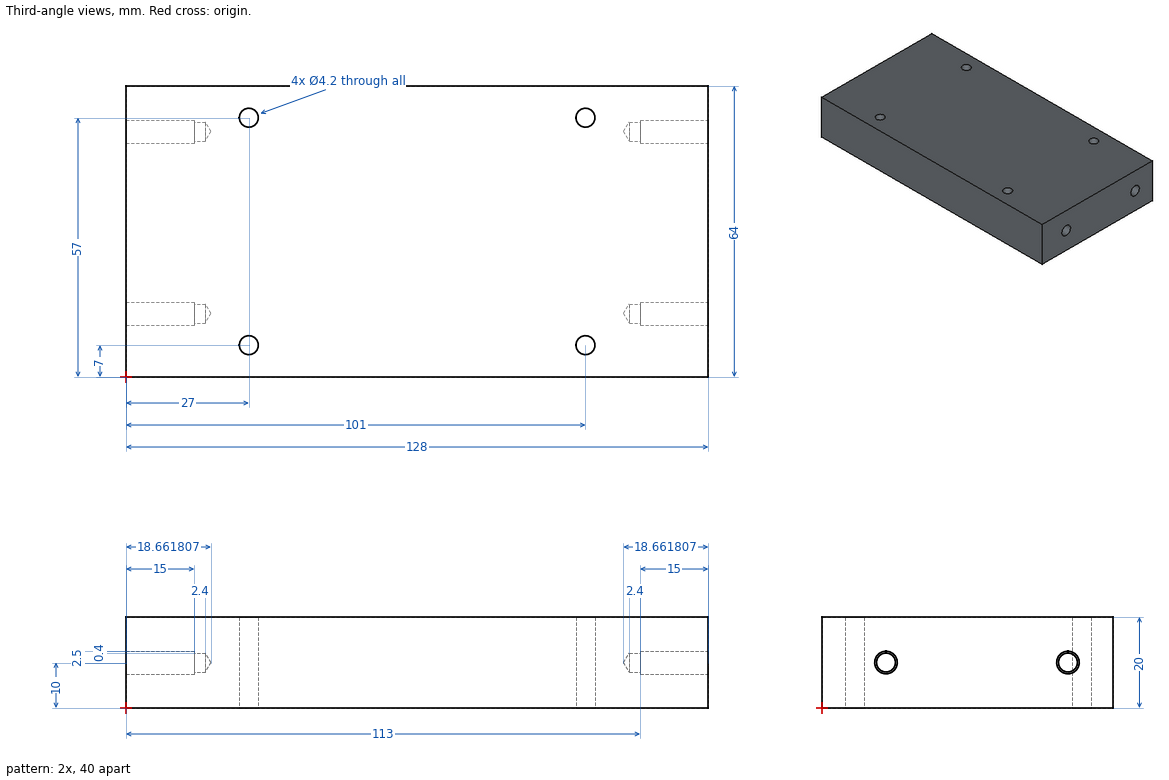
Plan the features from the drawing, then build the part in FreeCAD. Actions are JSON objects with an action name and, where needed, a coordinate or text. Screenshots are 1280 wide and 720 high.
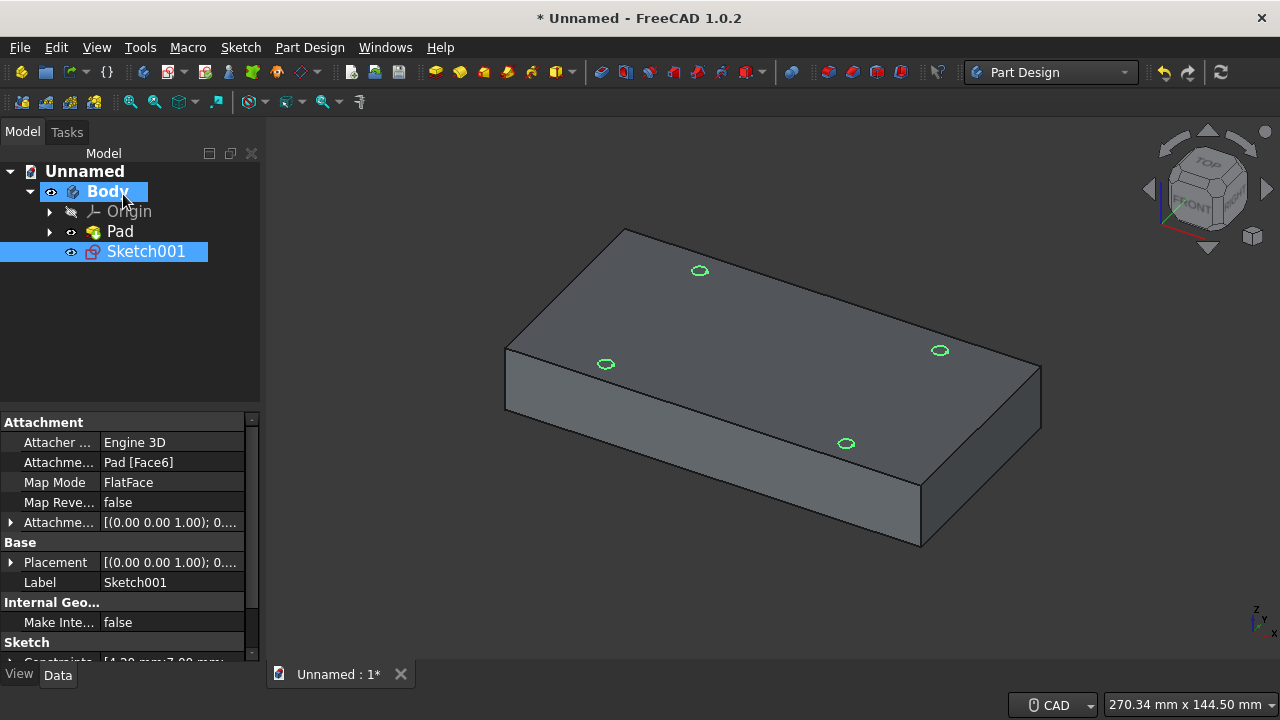
{"action": "left_click", "coordinate": [626, 72]}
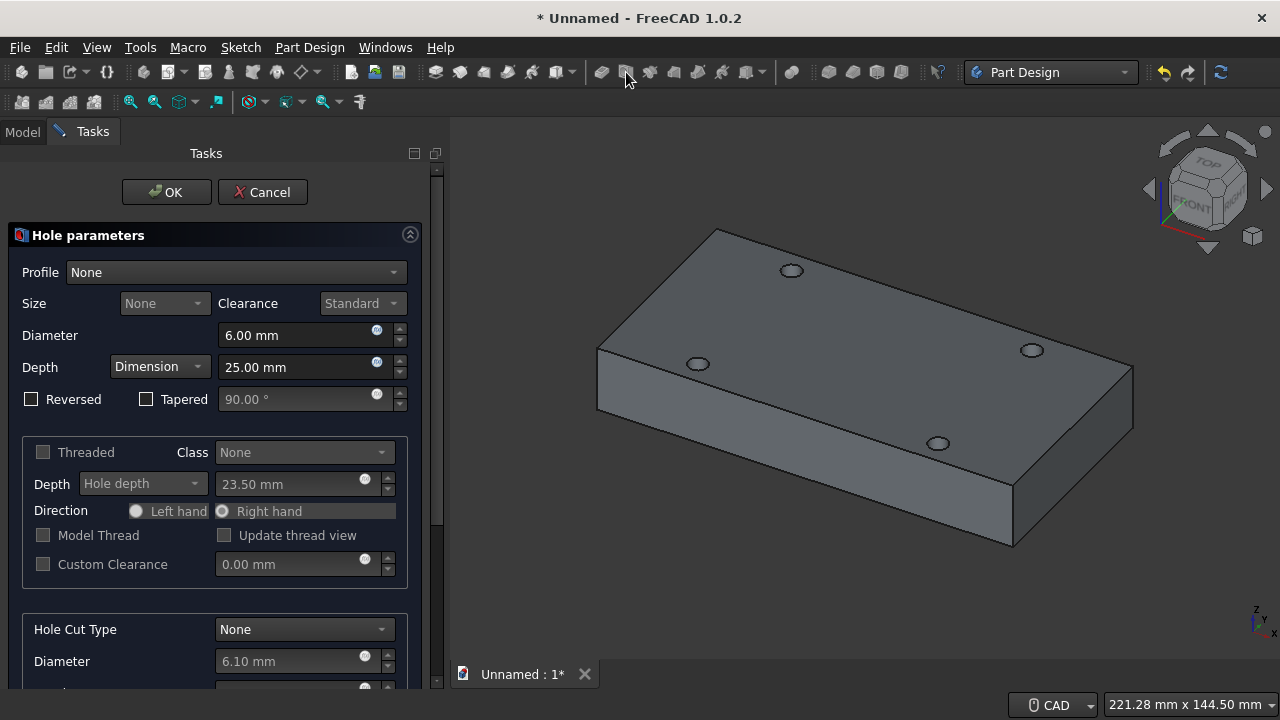
{"action": "triple_click", "coordinate": [305, 335]}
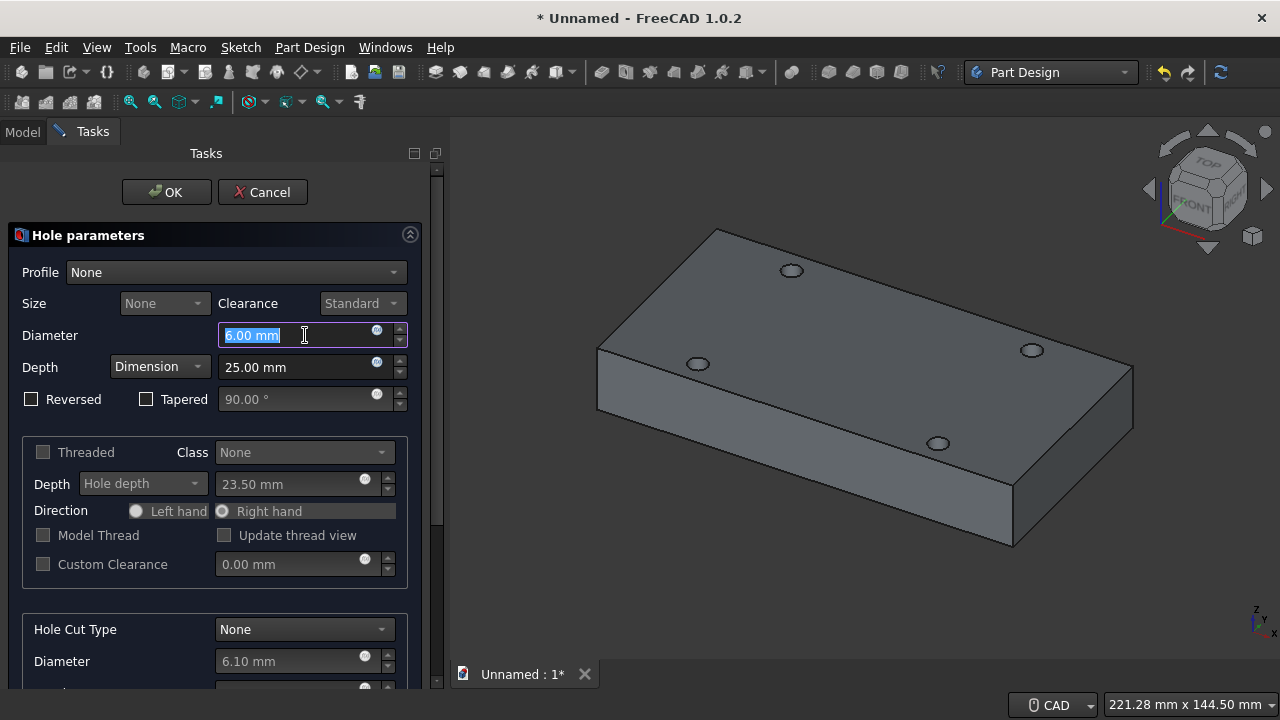
{"action": "type", "text": "4.2"}
{"action": "key", "text": "Tab"}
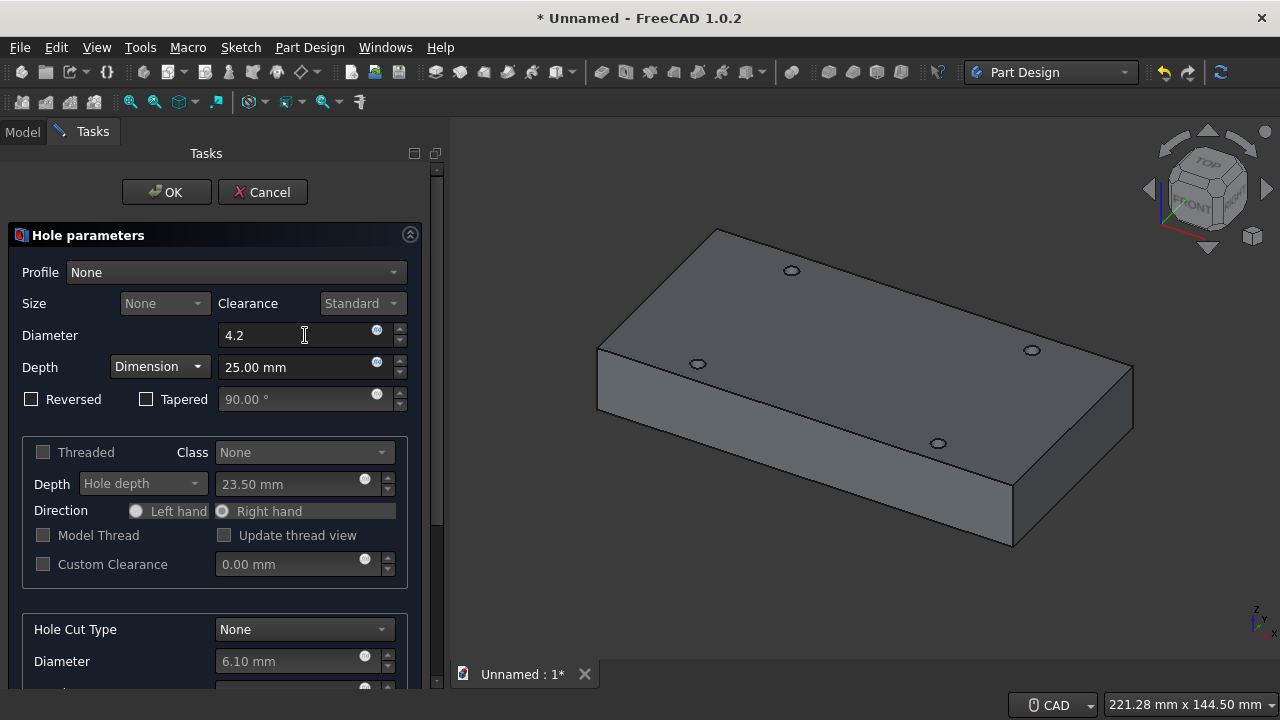
{"action": "left_click", "coordinate": [161, 366]}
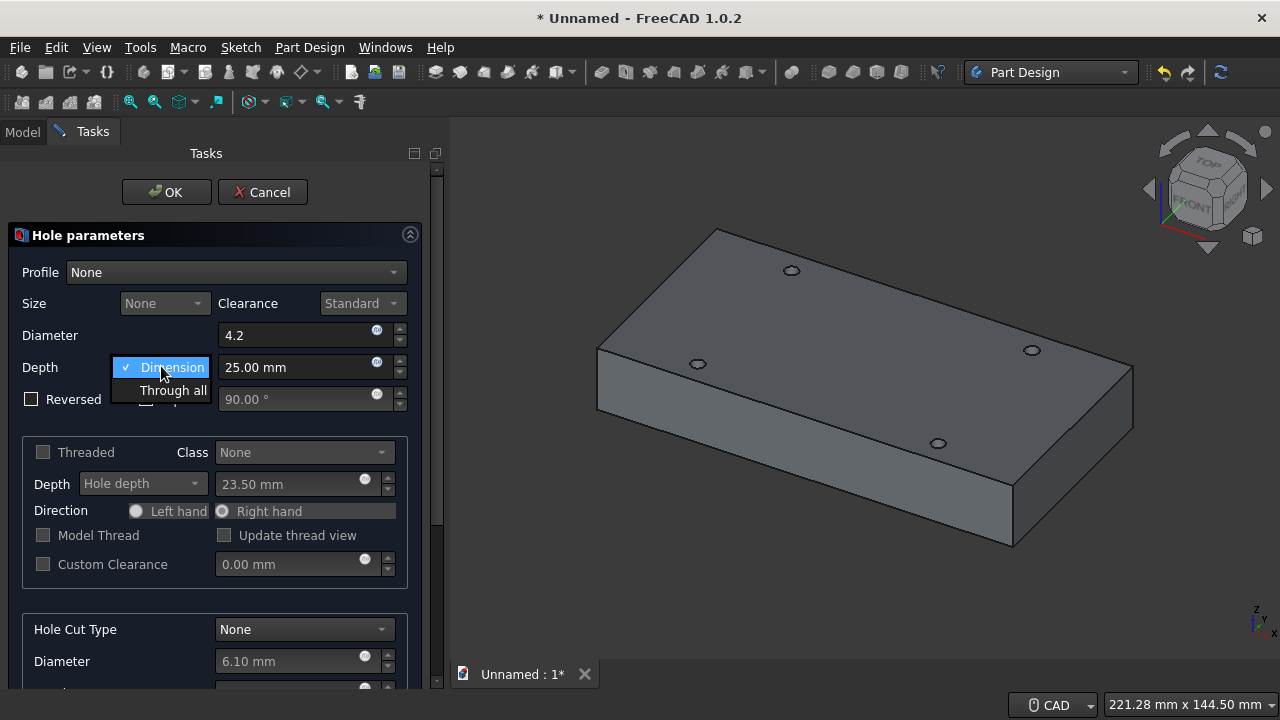
{"action": "left_click", "coordinate": [160, 390]}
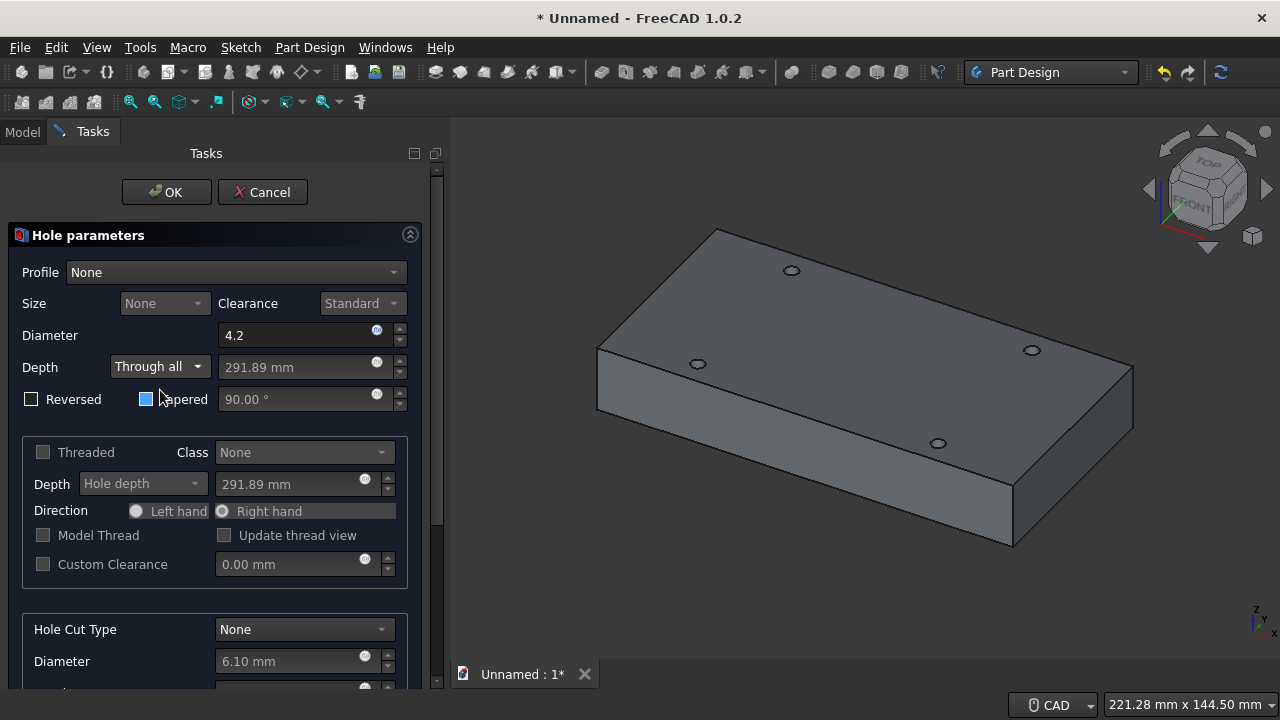
{"action": "left_click", "coordinate": [167, 192]}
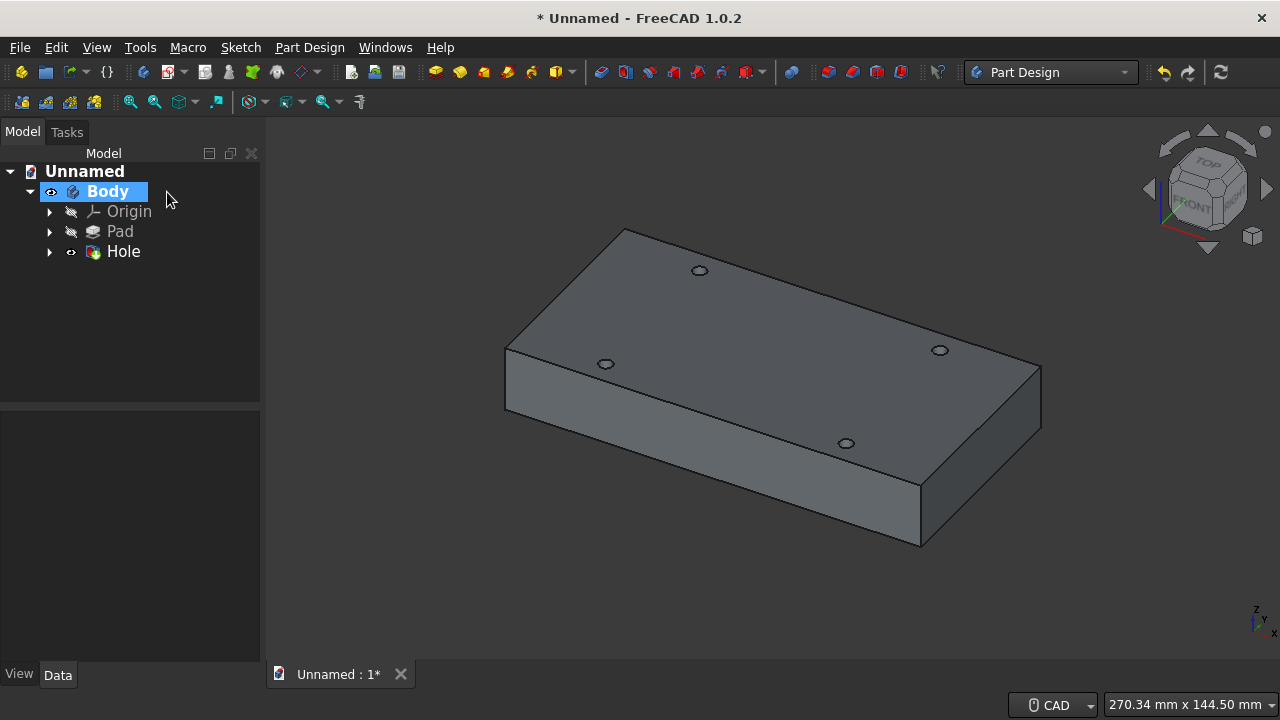
{"action": "left_click", "coordinate": [50, 212]}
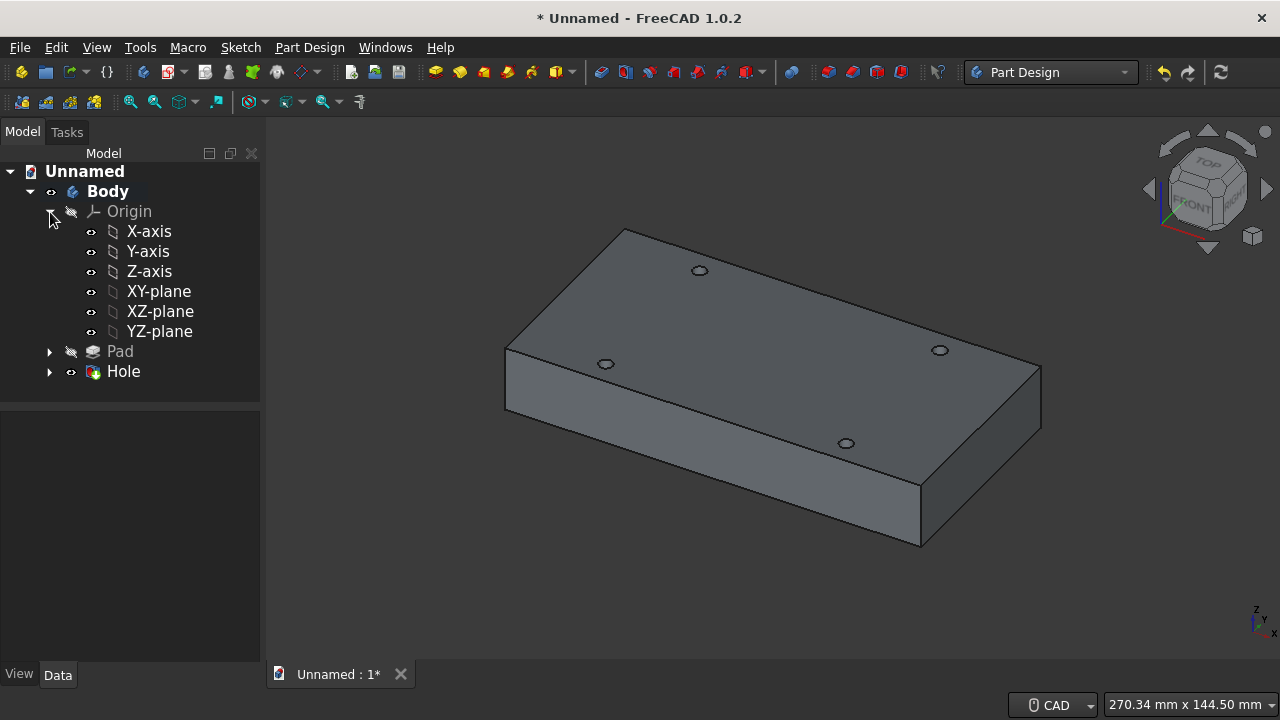
{"action": "left_click", "coordinate": [136, 312]}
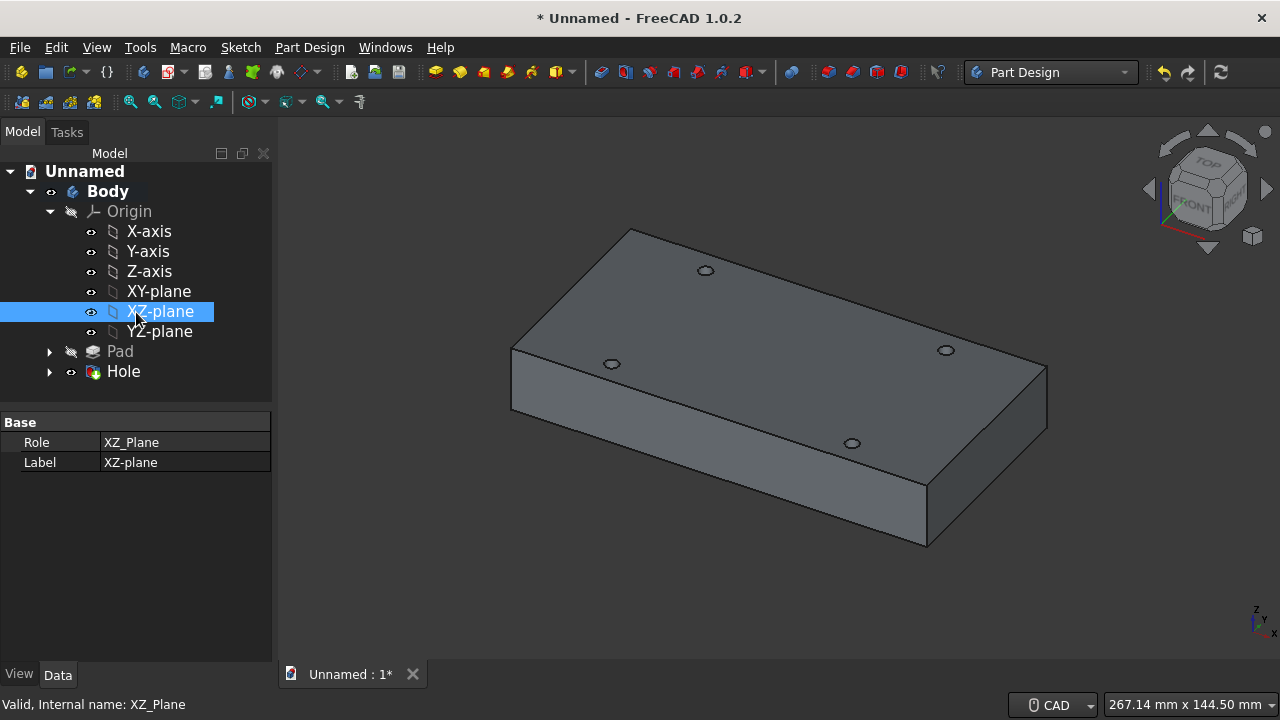
{"action": "left_click", "coordinate": [302, 72]}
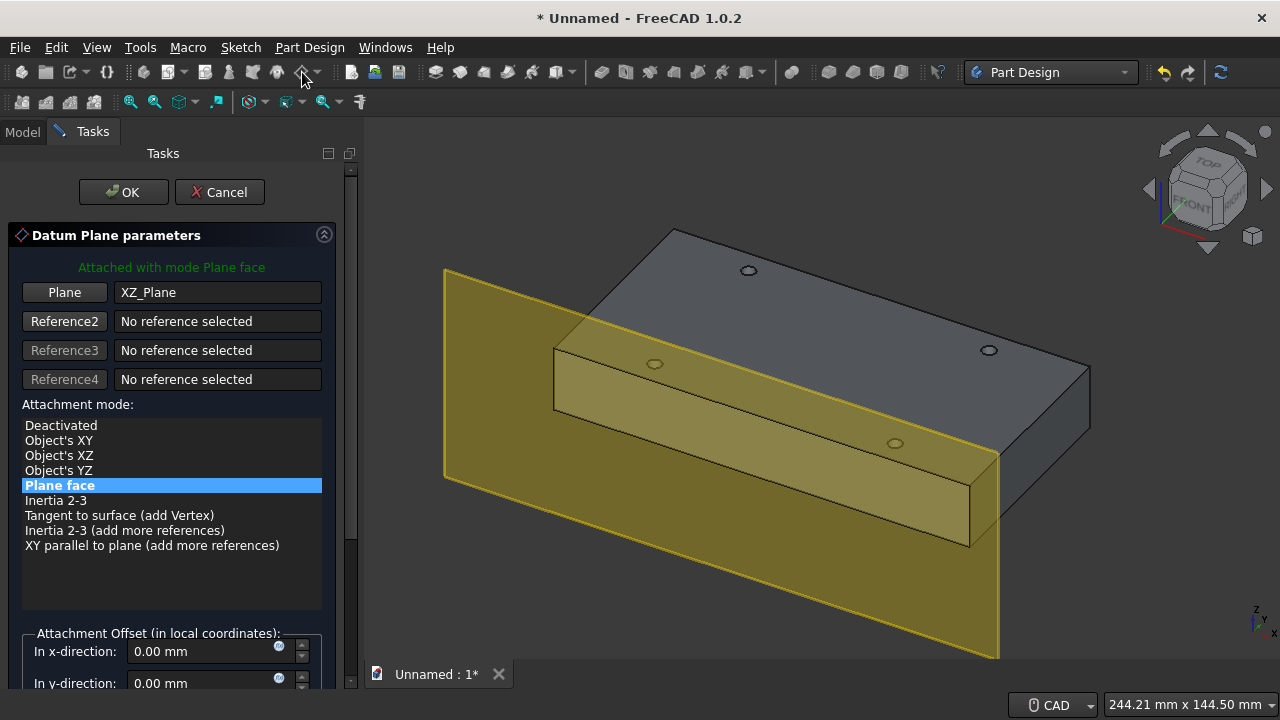
{"action": "scroll", "coordinate": [351, 426], "scroll_direction": "down", "scroll_amount": 2}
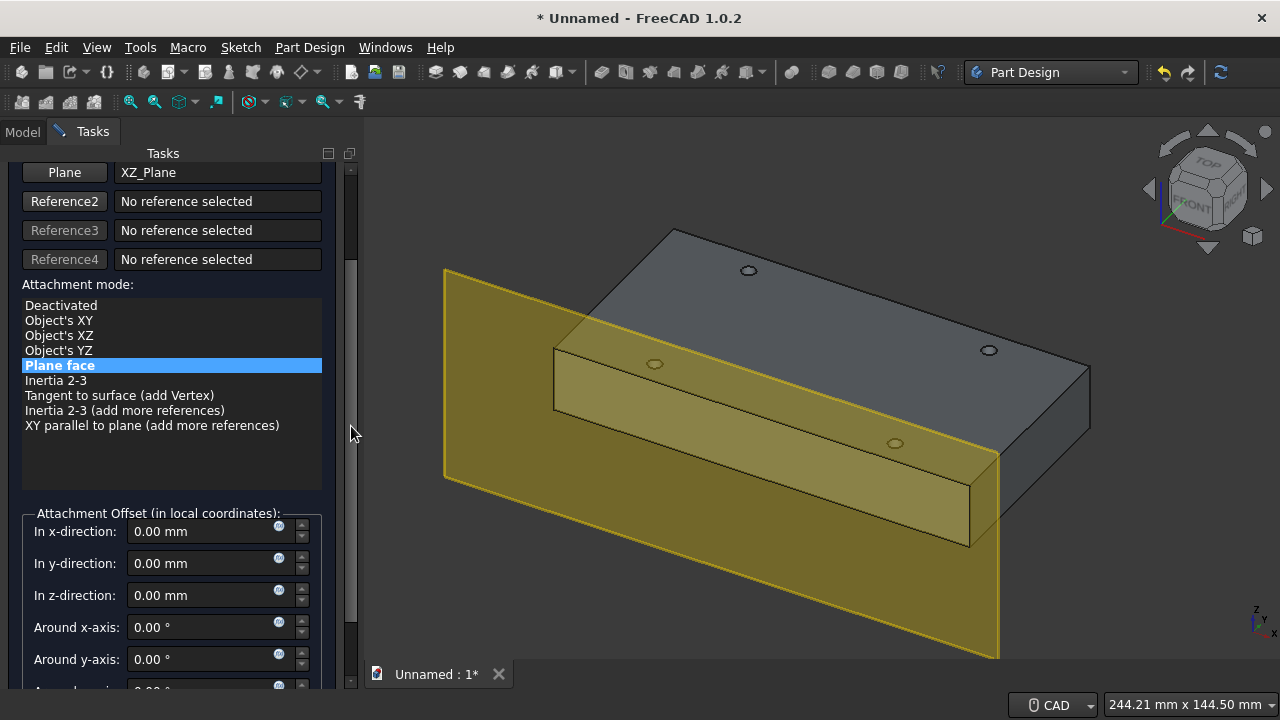
{"action": "triple_click", "coordinate": [210, 595]}